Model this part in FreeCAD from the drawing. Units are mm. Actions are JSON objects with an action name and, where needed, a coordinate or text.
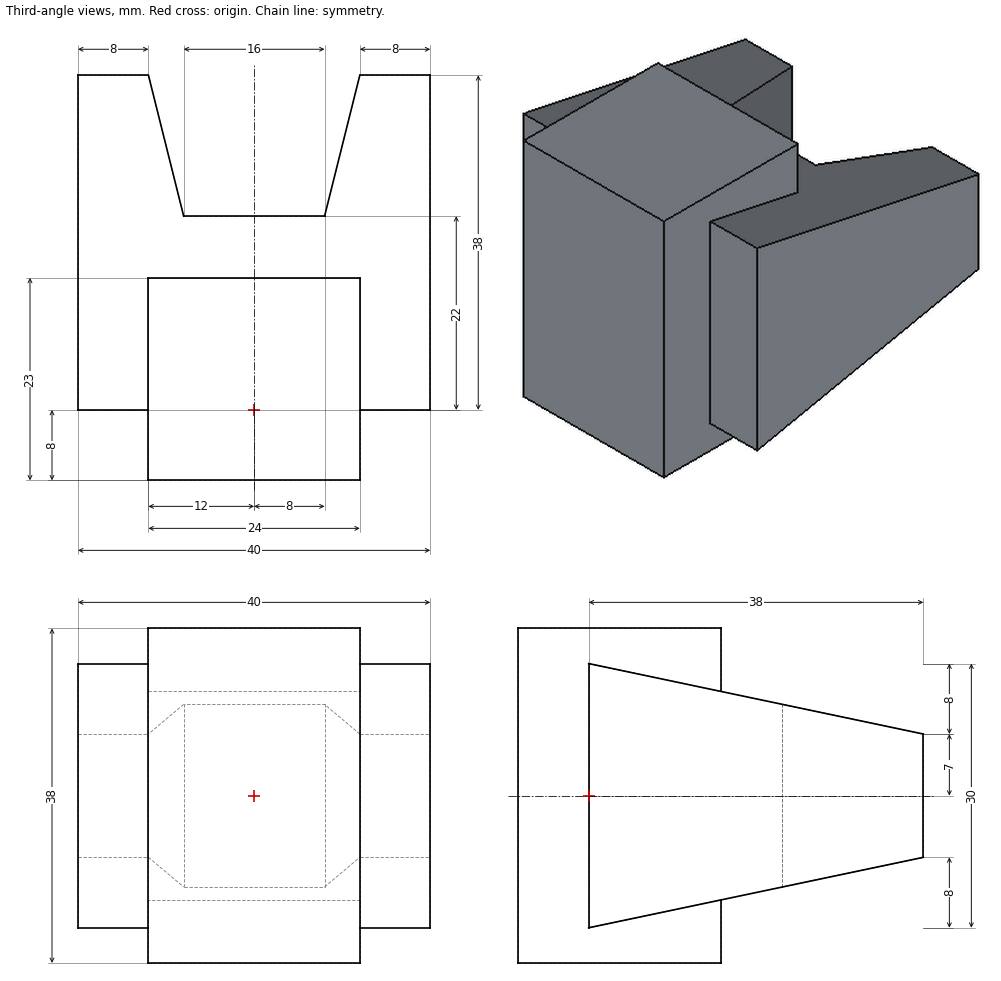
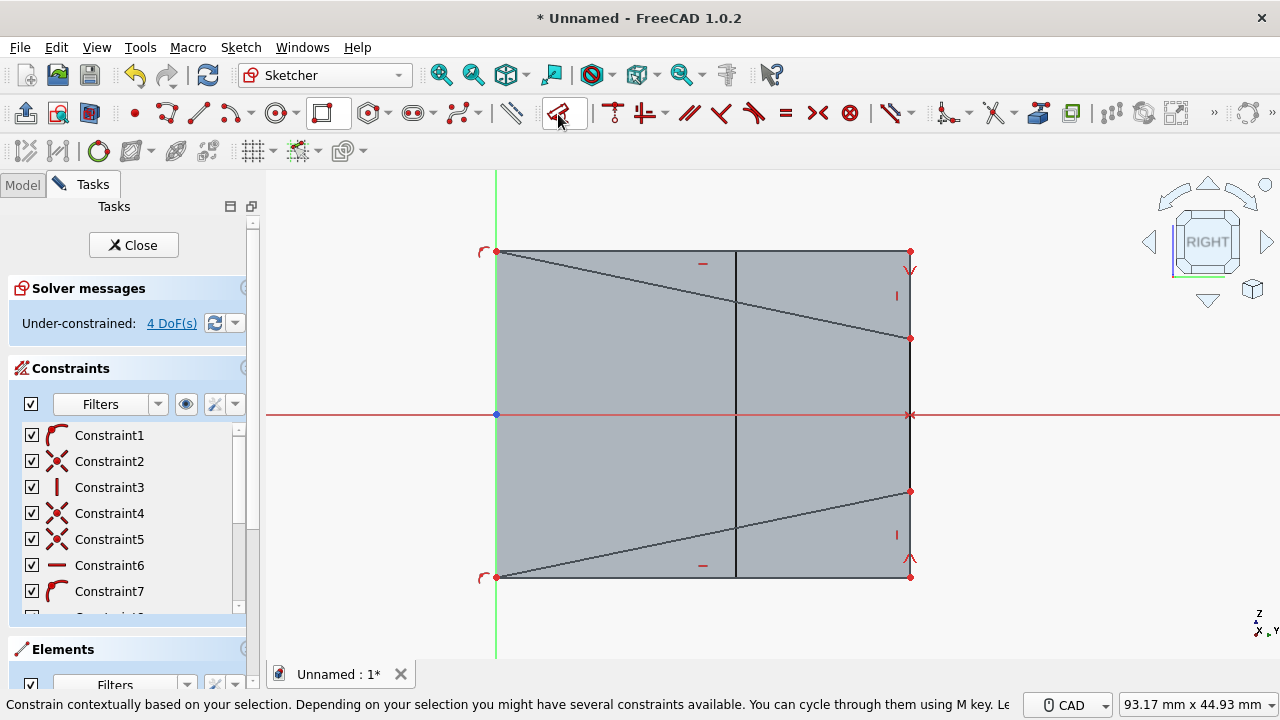
{"action": "left_click", "coordinate": [910, 313]}
{"action": "left_click", "coordinate": [944, 295]}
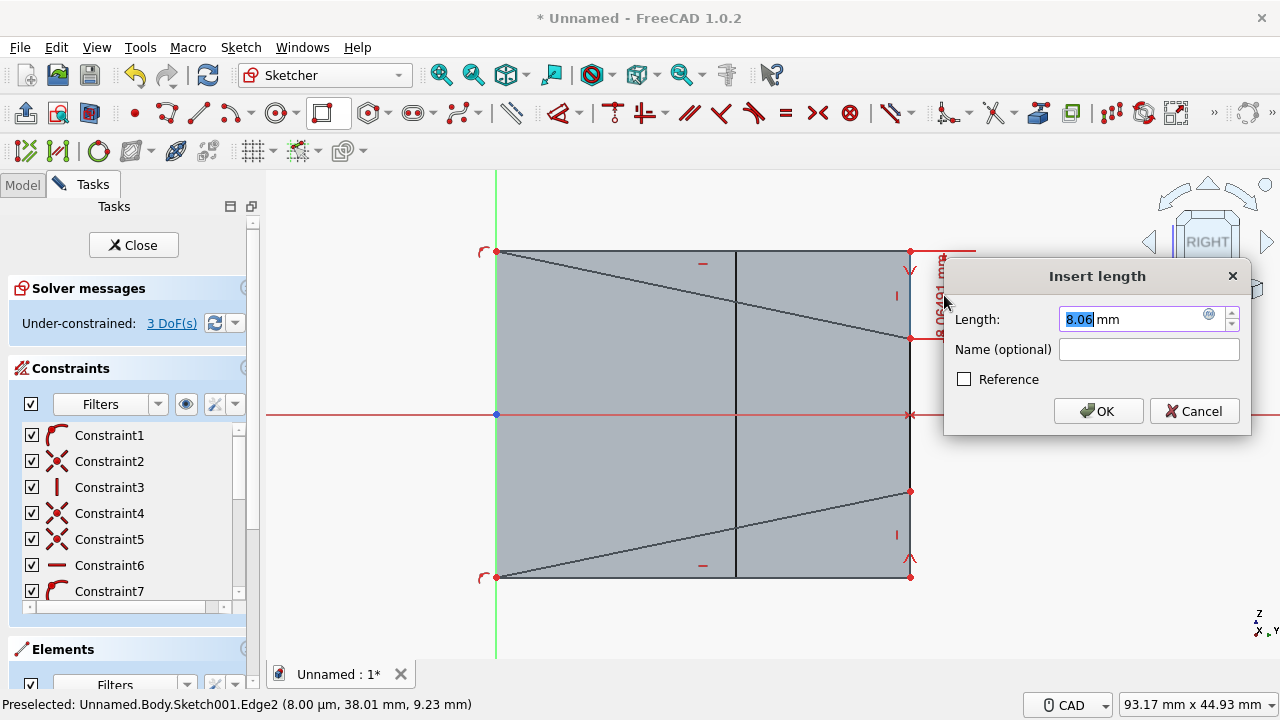
{"action": "type", "text": "8"}
{"action": "key", "text": "Return"}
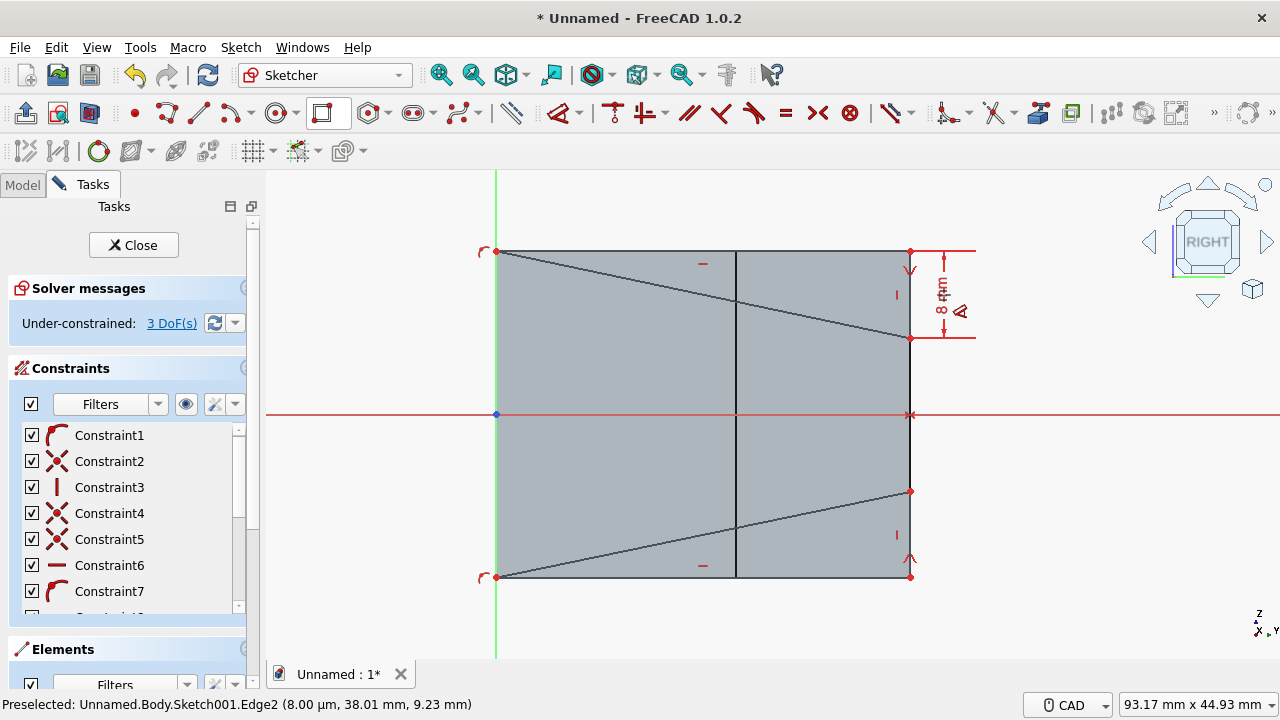
{"action": "left_click", "coordinate": [910, 552]}
{"action": "left_click", "coordinate": [944, 535]}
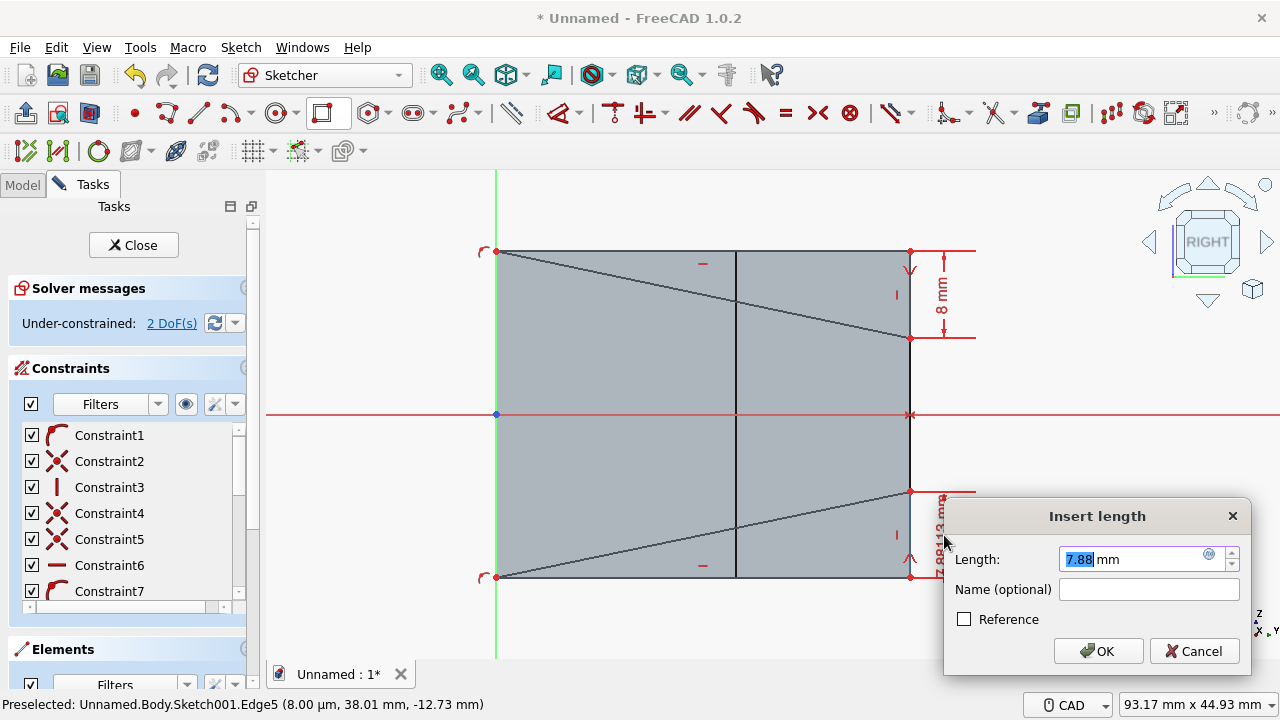
{"action": "type", "text": "8"}
{"action": "key", "text": "Return"}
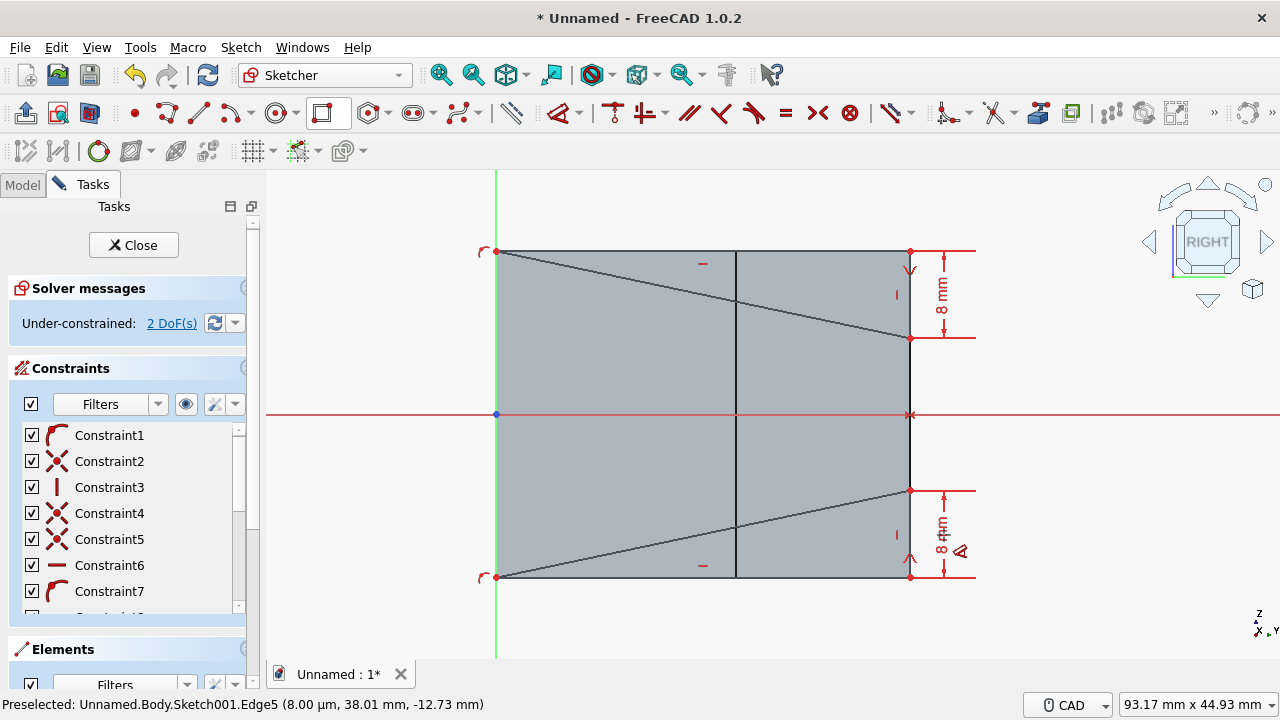
{"action": "left_click", "coordinate": [786, 251]}
{"action": "left_click", "coordinate": [703, 217]}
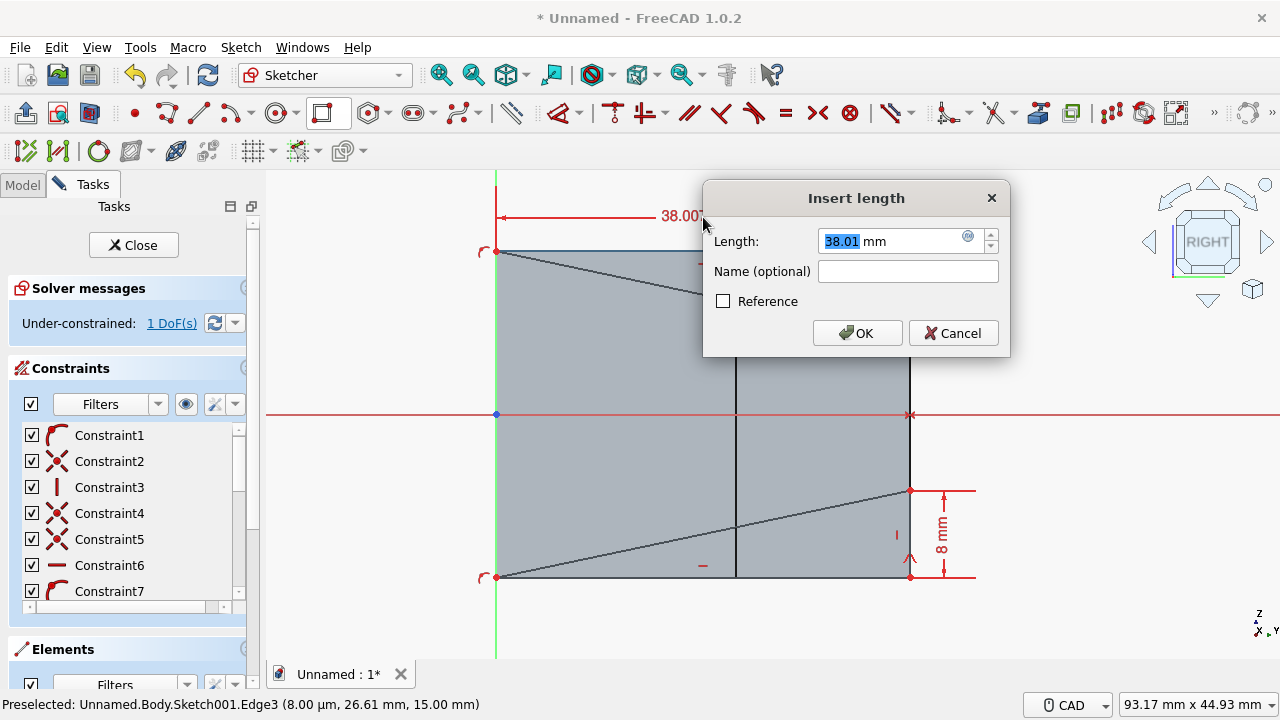
{"action": "type", "text": "38"}
{"action": "key", "text": "Return"}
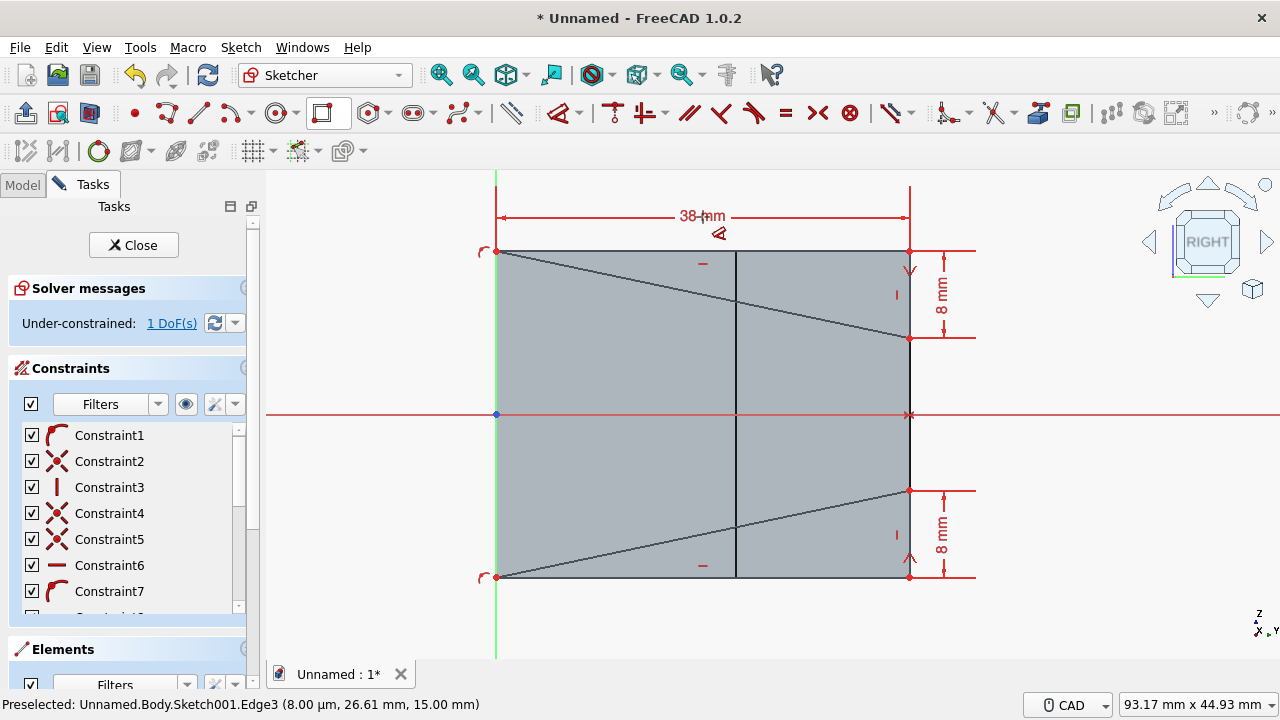
{"action": "left_click", "coordinate": [910, 338]}
{"action": "left_click", "coordinate": [944, 376]}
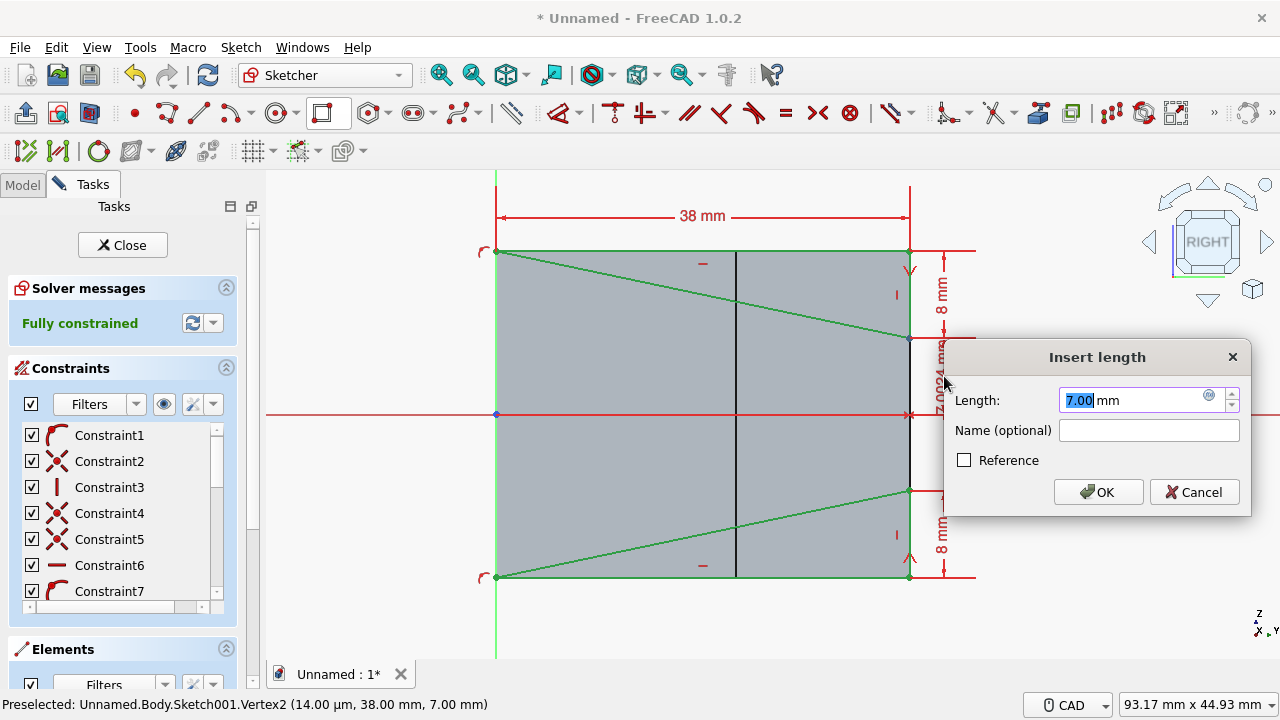
{"action": "type", "text": "7"}
{"action": "key", "text": "Return"}
{"action": "key", "text": "Escape"}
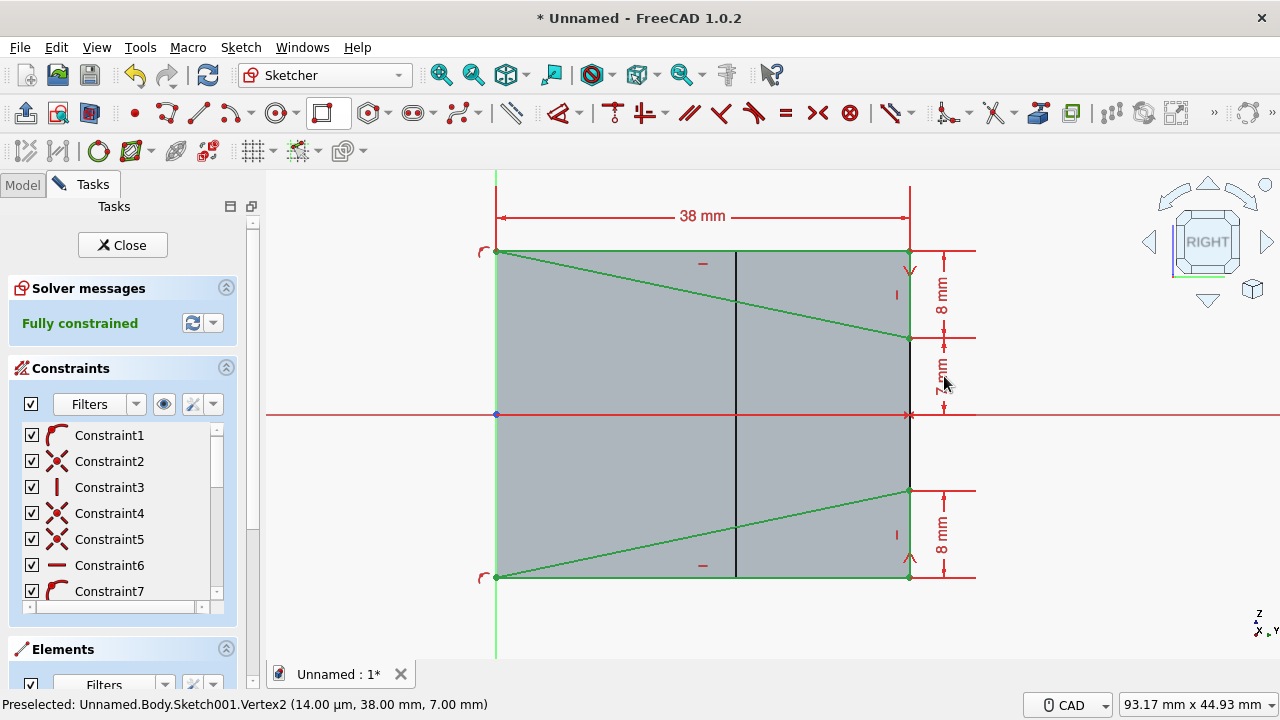
{"action": "left_click", "coordinate": [123, 245]}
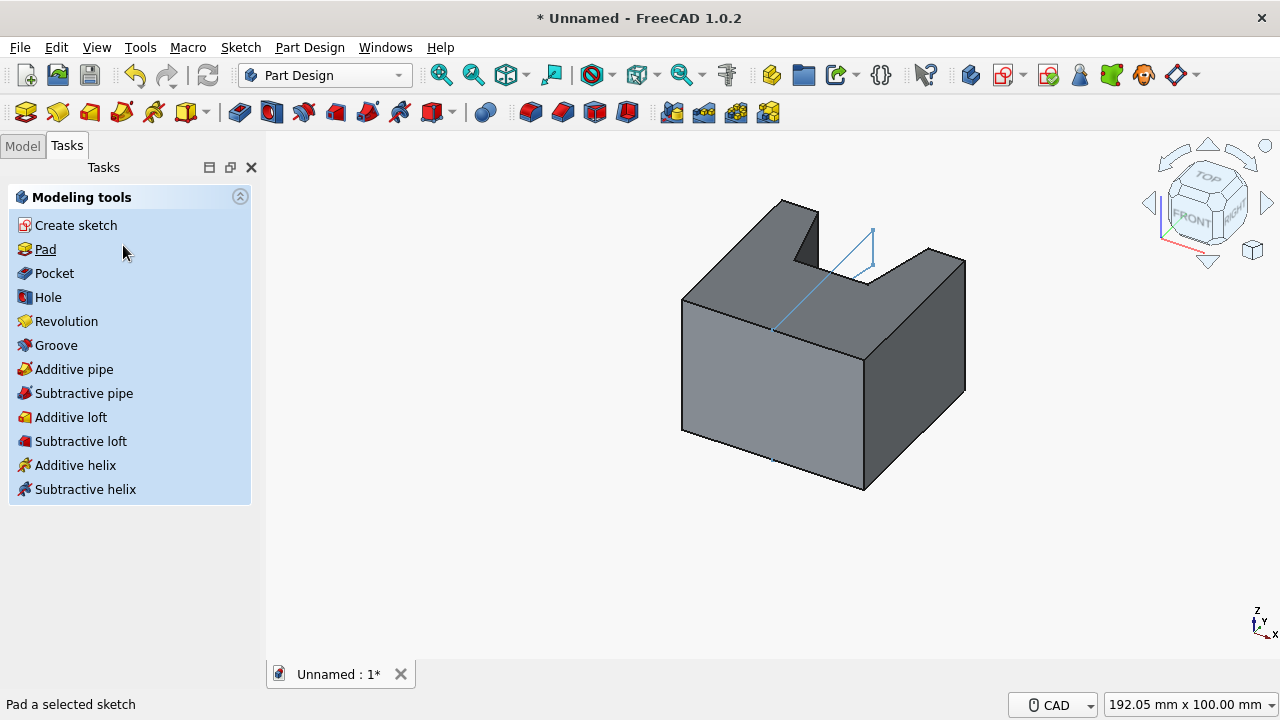
{"action": "left_click", "coordinate": [240, 112]}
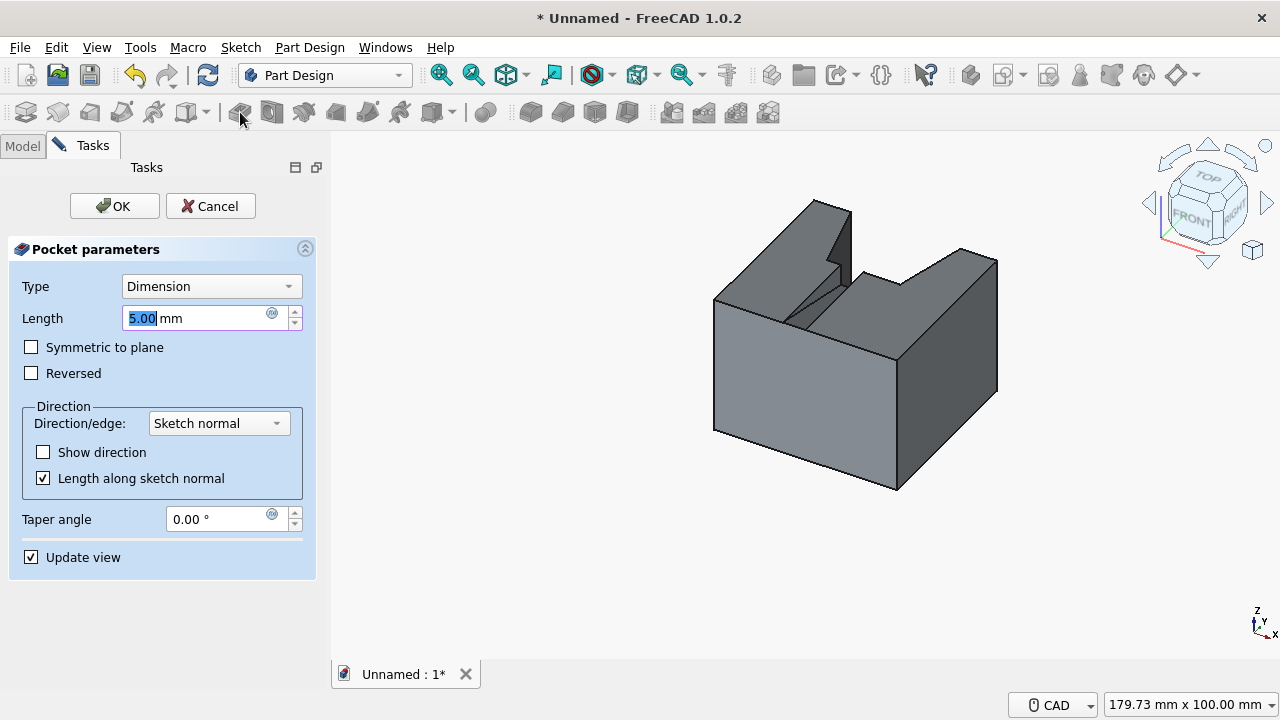
{"action": "type", "text": "40"}
{"action": "key", "text": "Tab"}